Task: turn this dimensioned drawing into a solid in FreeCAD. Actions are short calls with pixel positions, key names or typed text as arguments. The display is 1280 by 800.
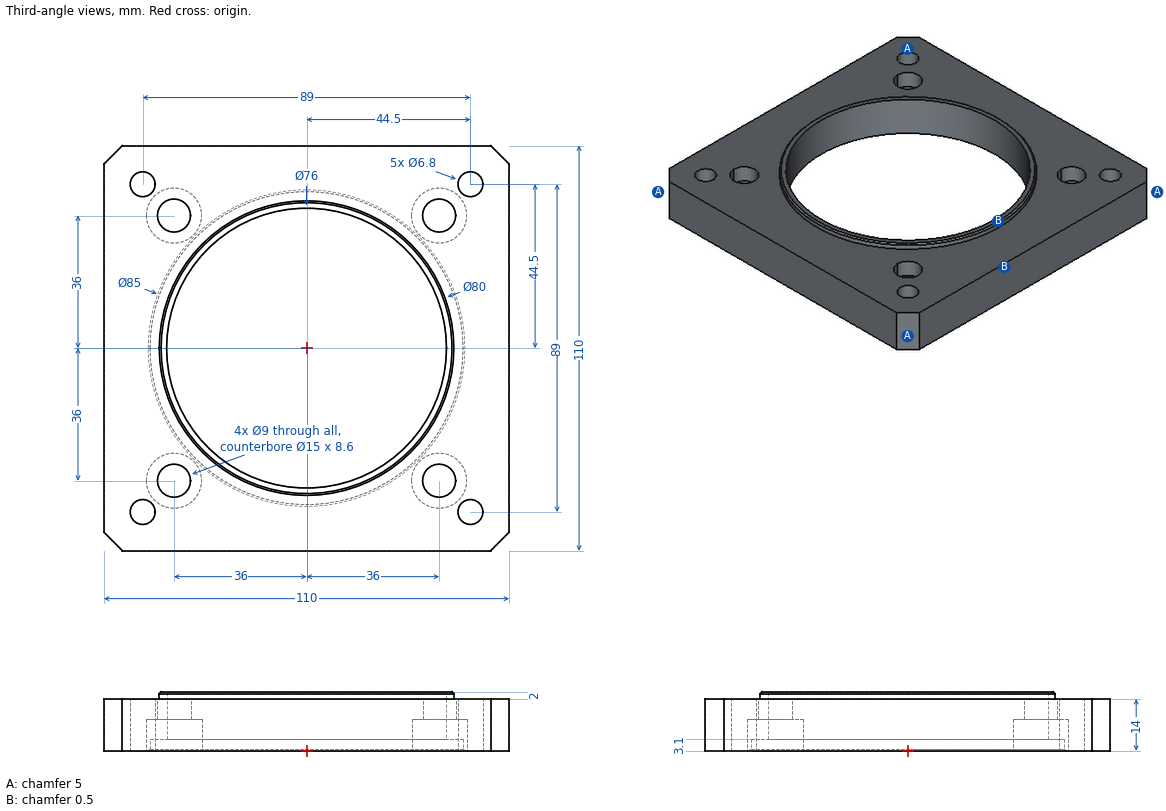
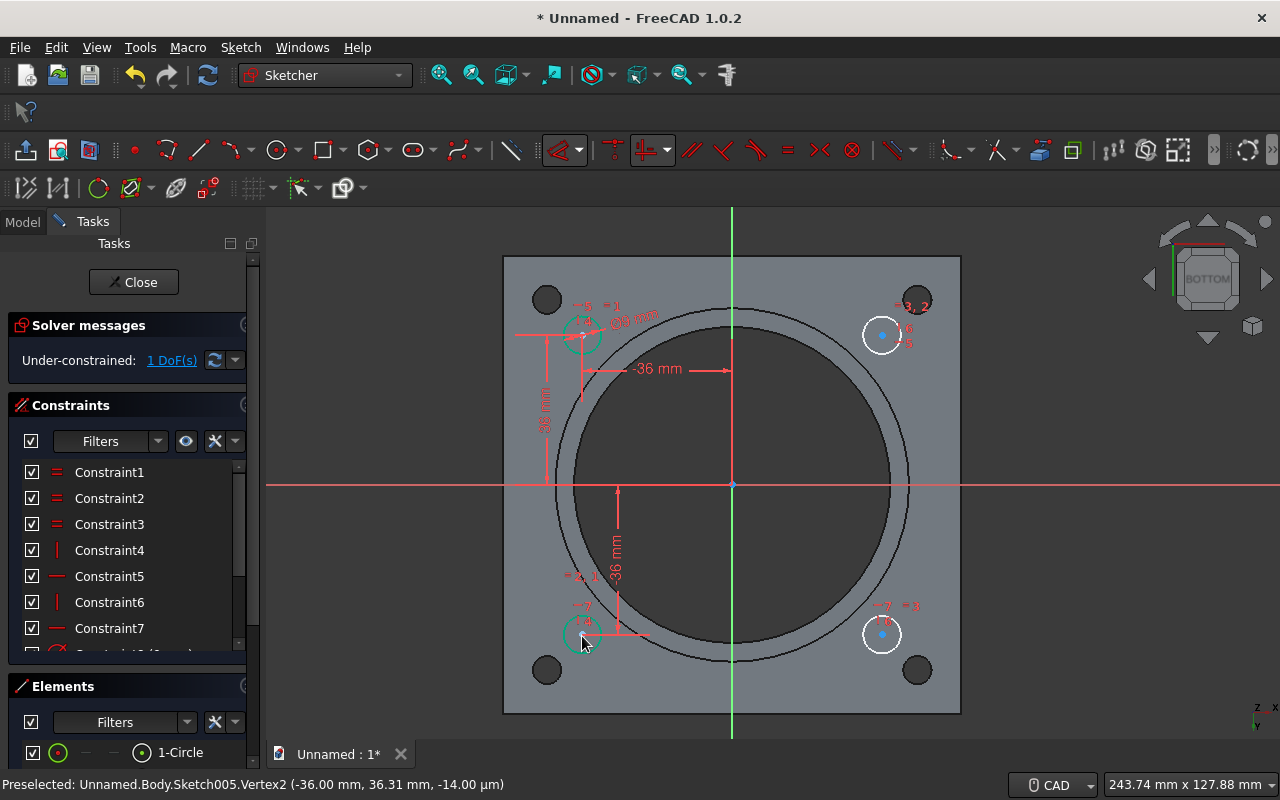
click(882, 335)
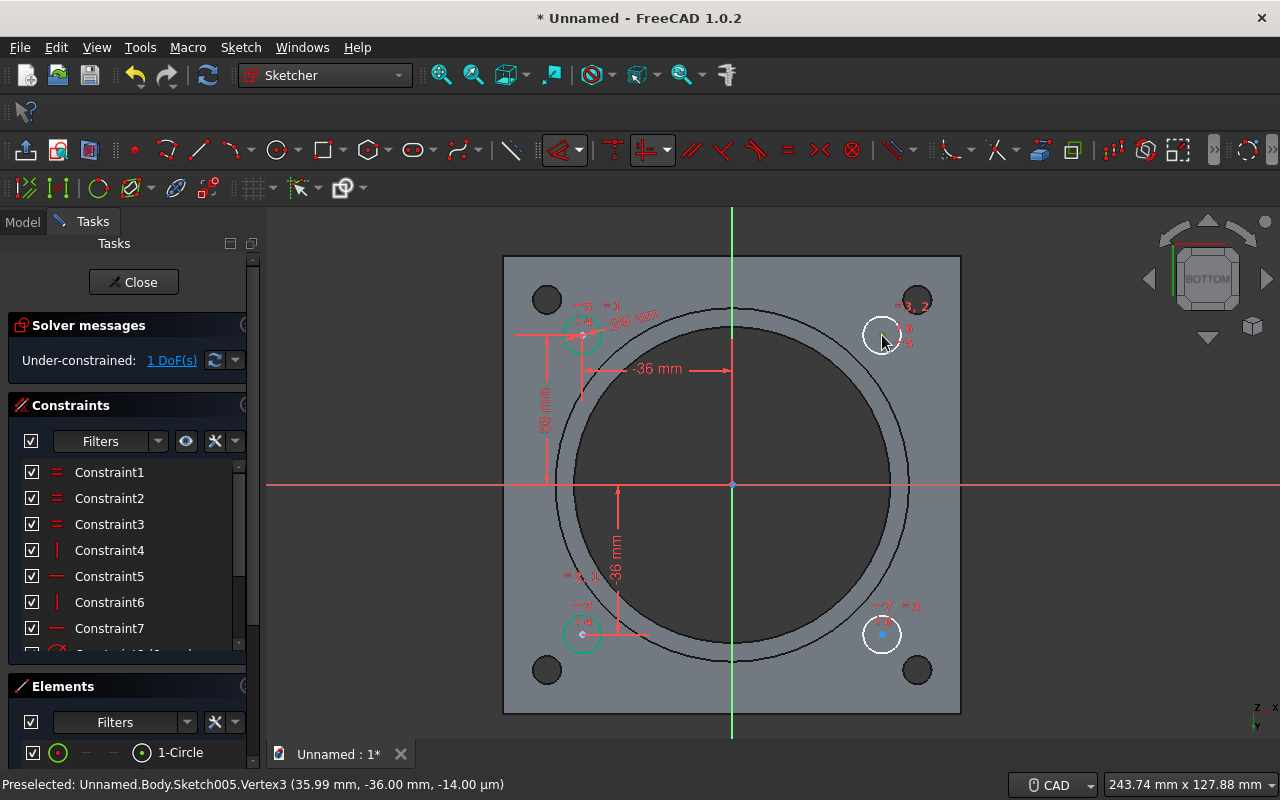
key(l)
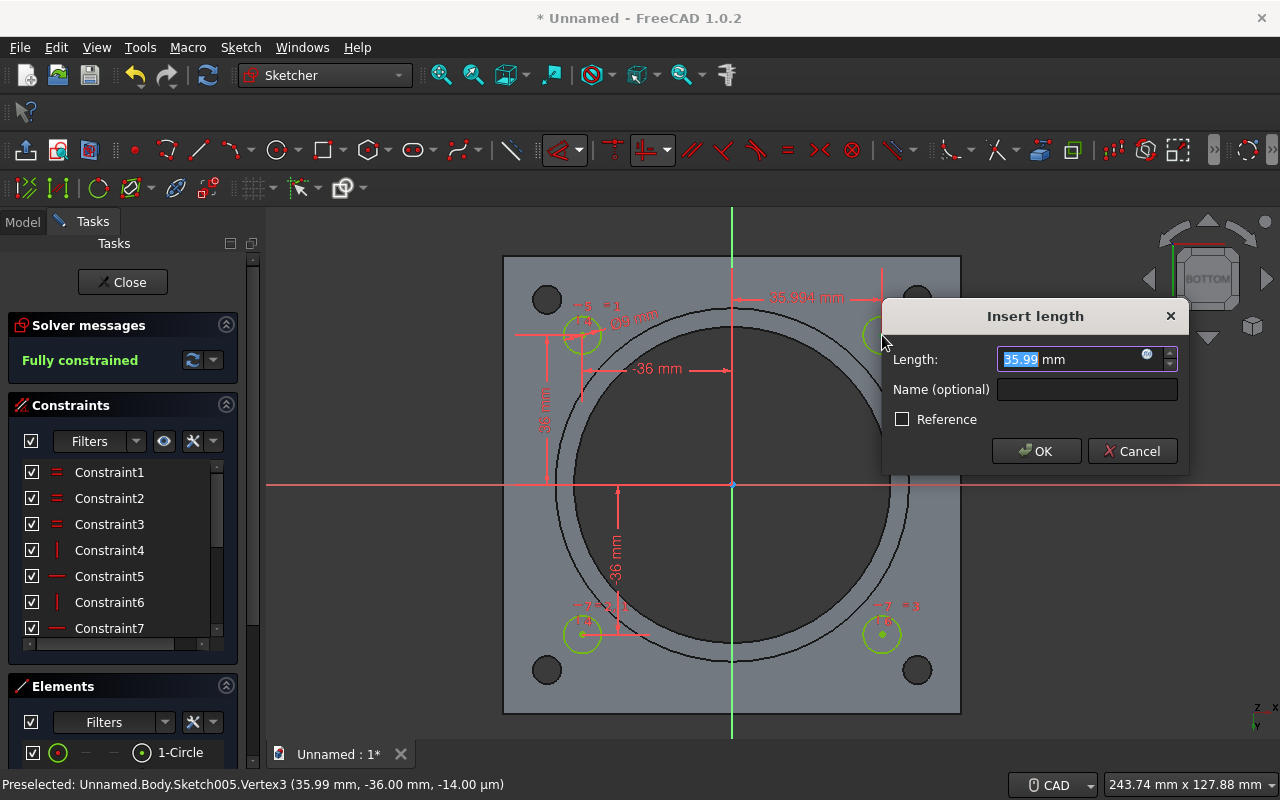
text(36)
key(Return)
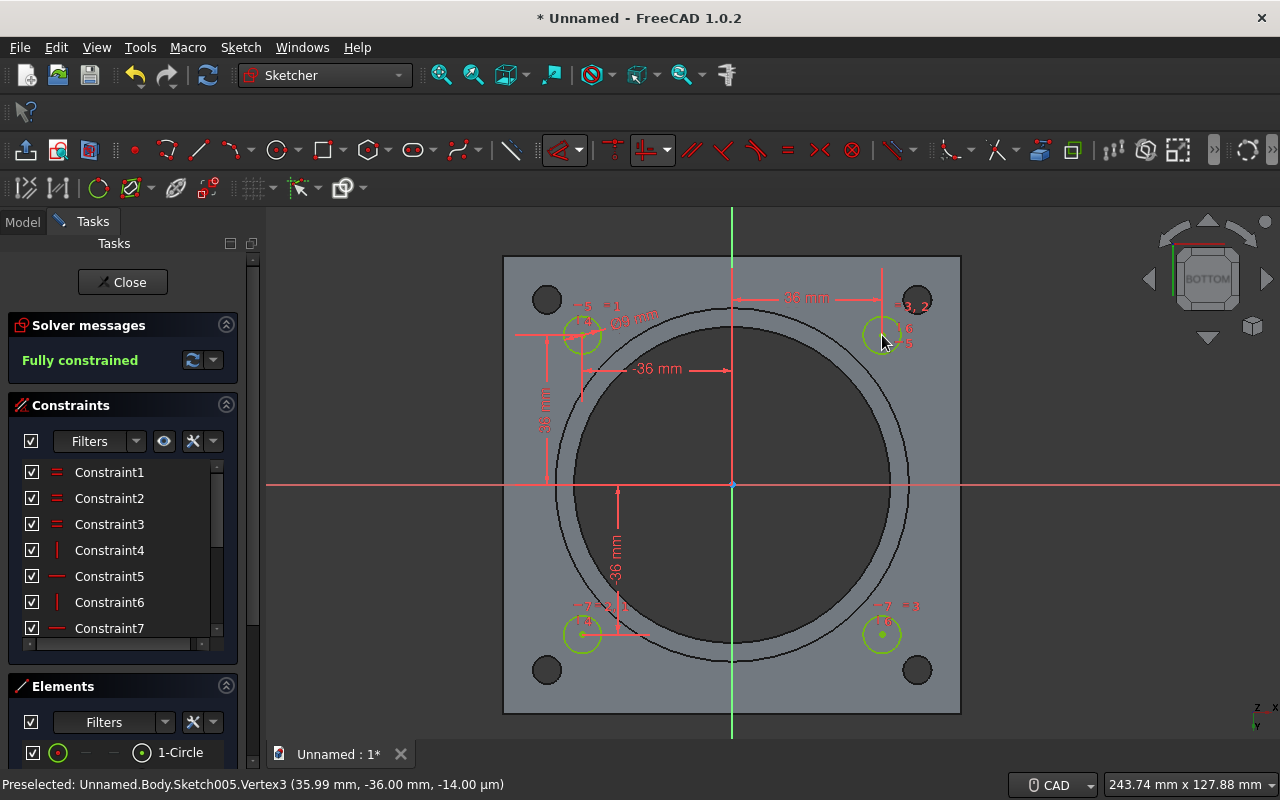
click(123, 282)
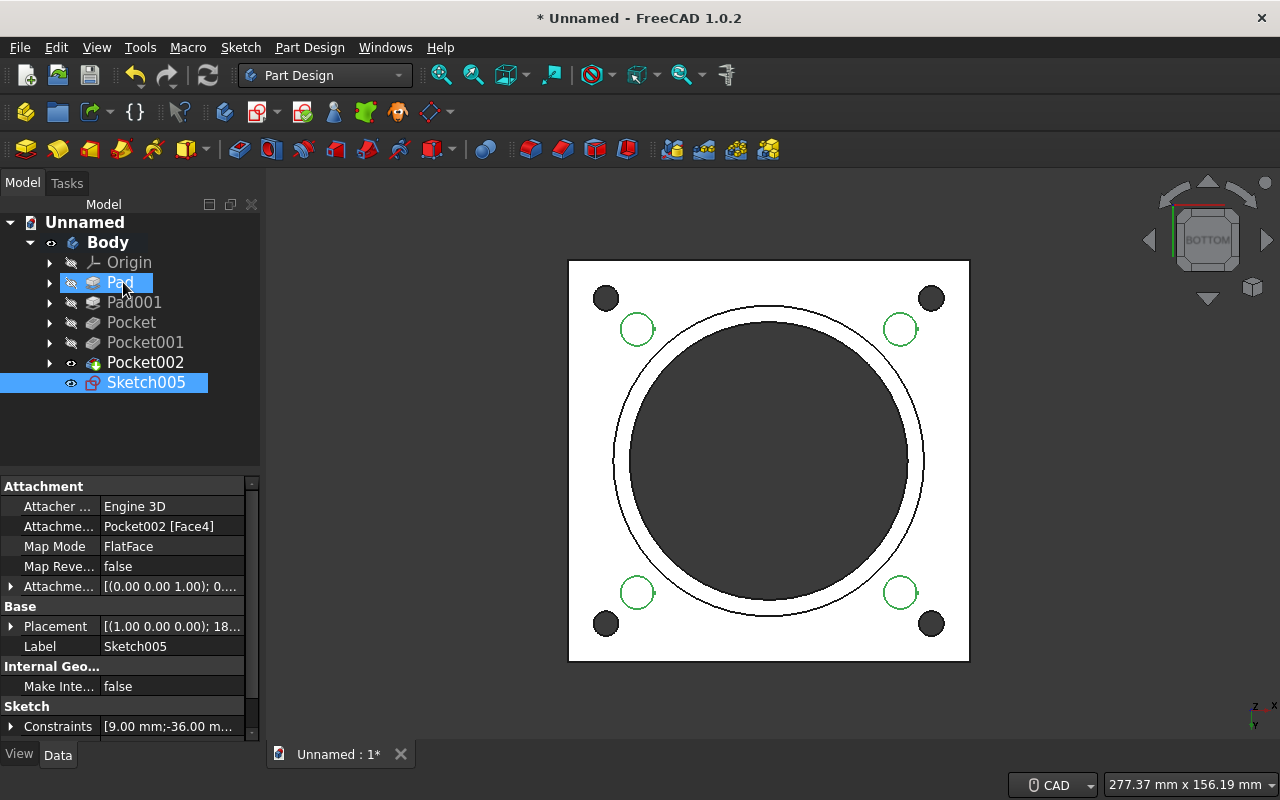
click(272, 150)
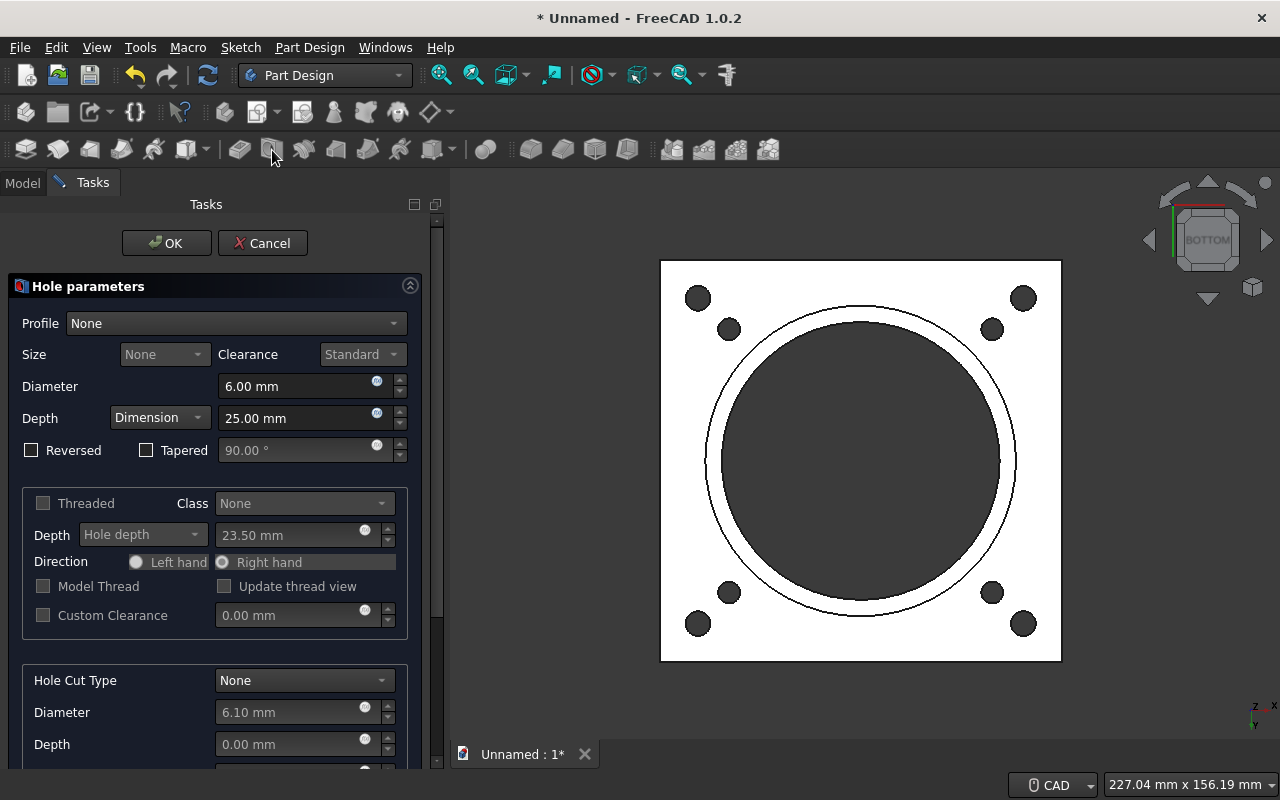
triple_click(305, 386)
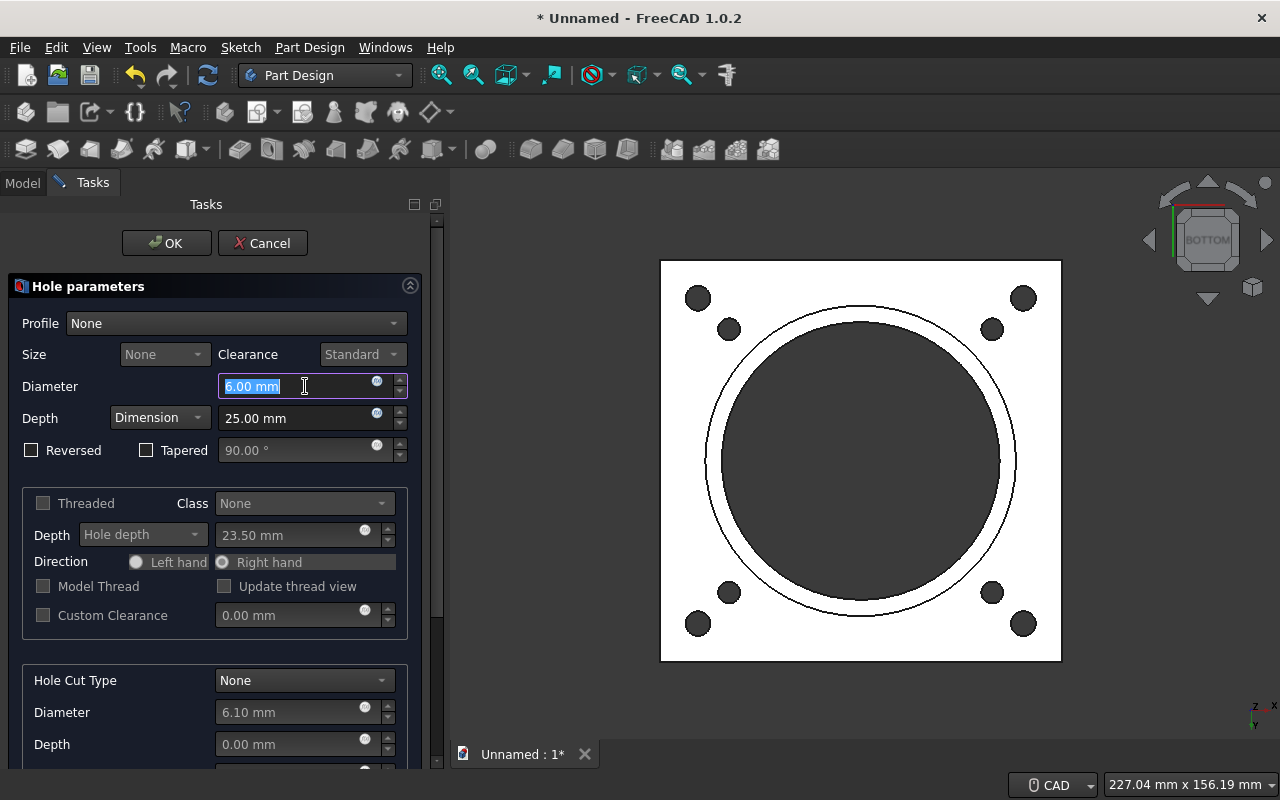
text(9)
key(Tab)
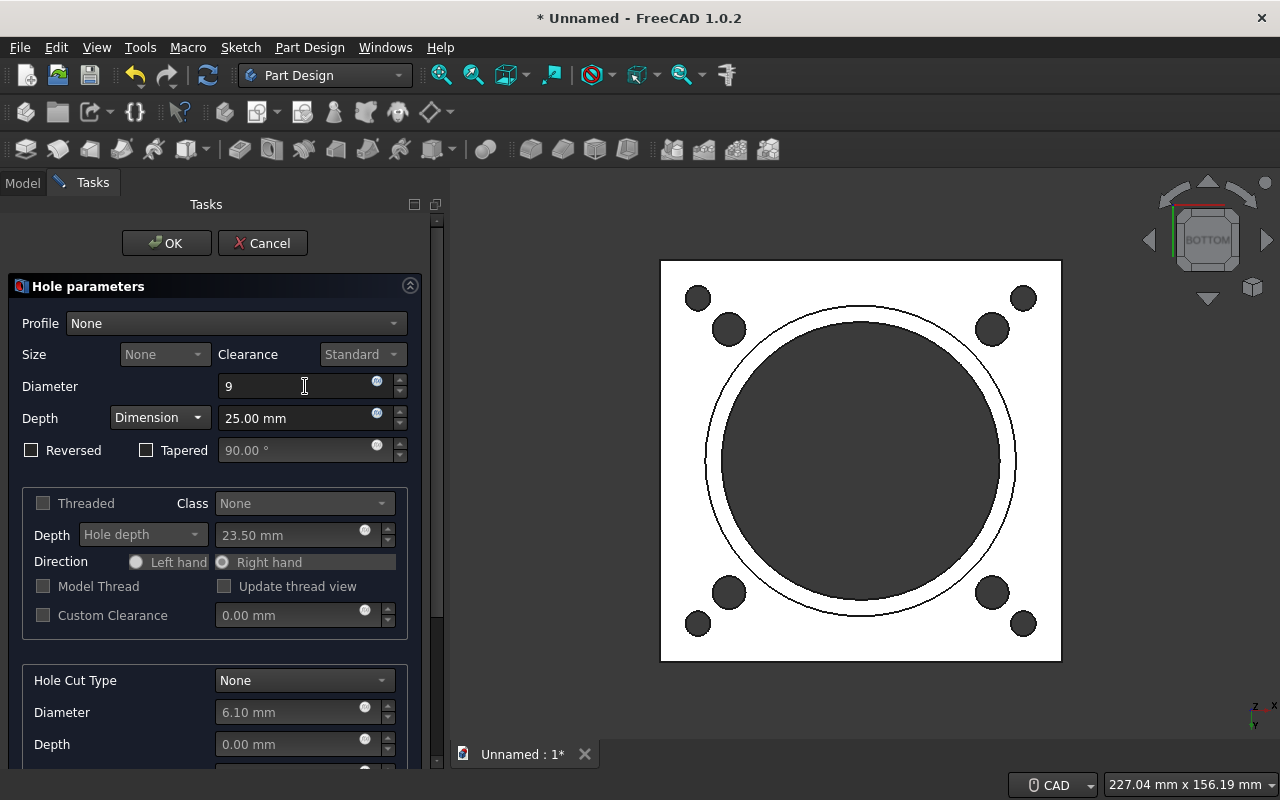
click(161, 418)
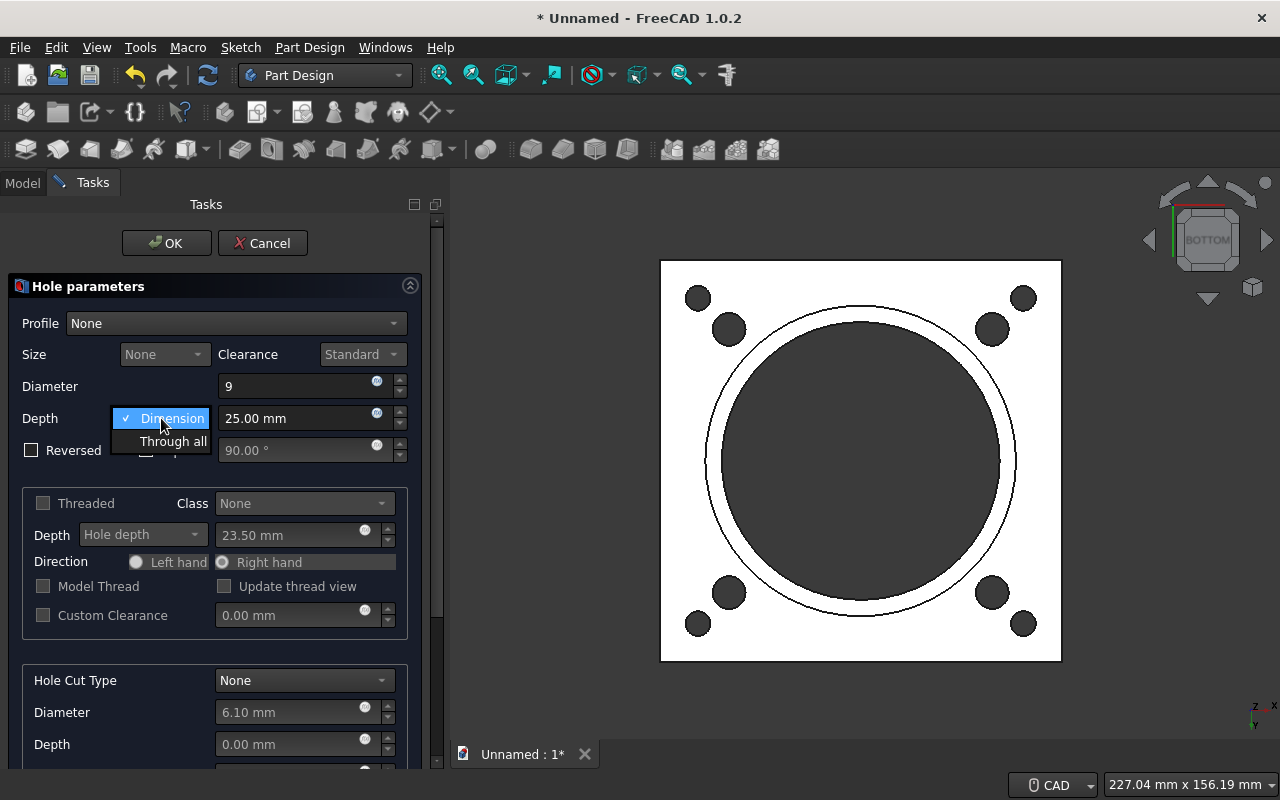
click(160, 442)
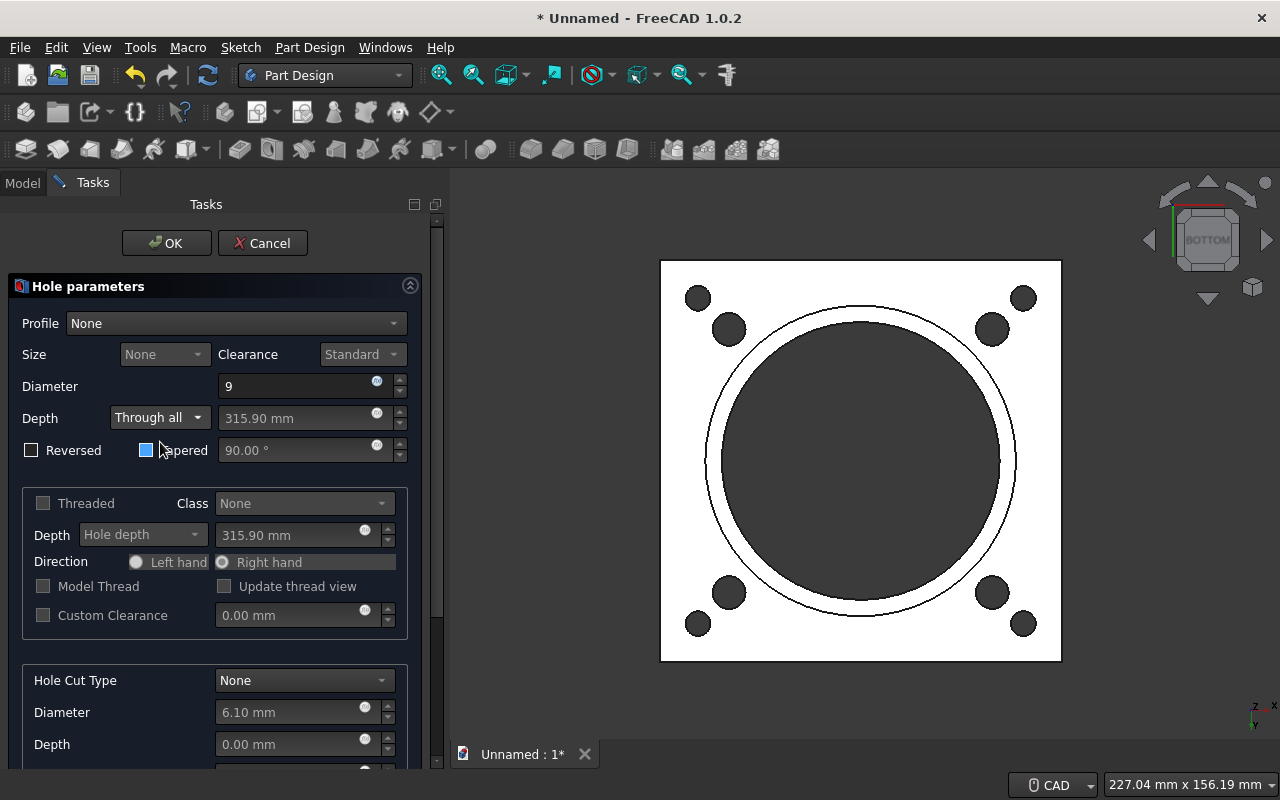
click(306, 680)